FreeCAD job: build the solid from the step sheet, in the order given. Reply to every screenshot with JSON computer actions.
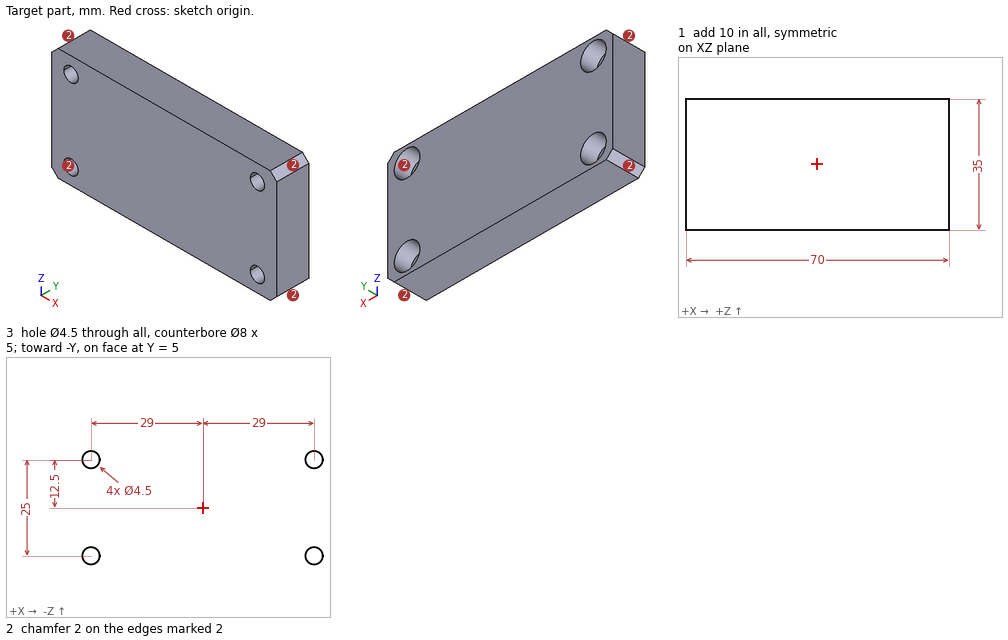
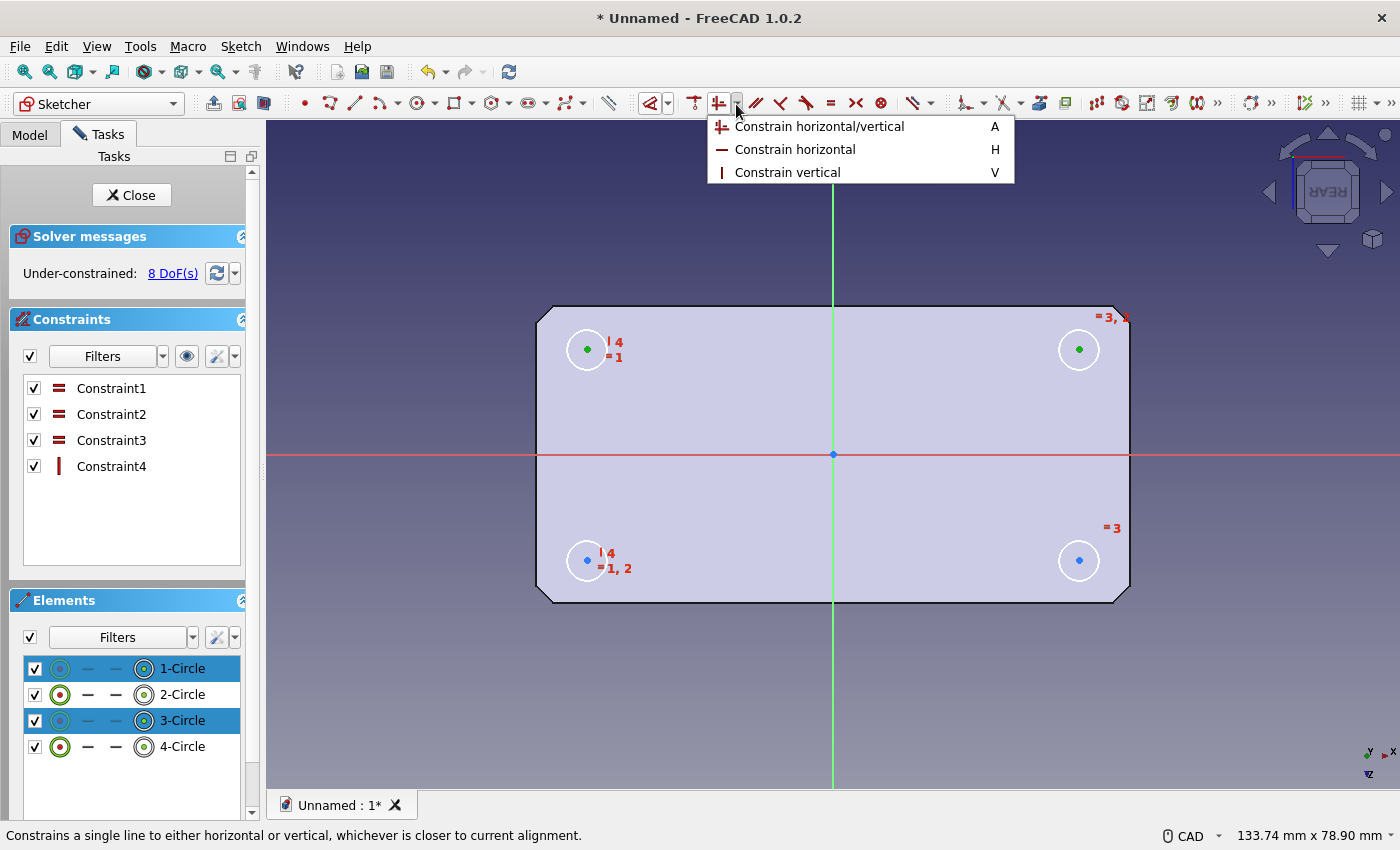
{"action": "left_click", "coordinate": [861, 150]}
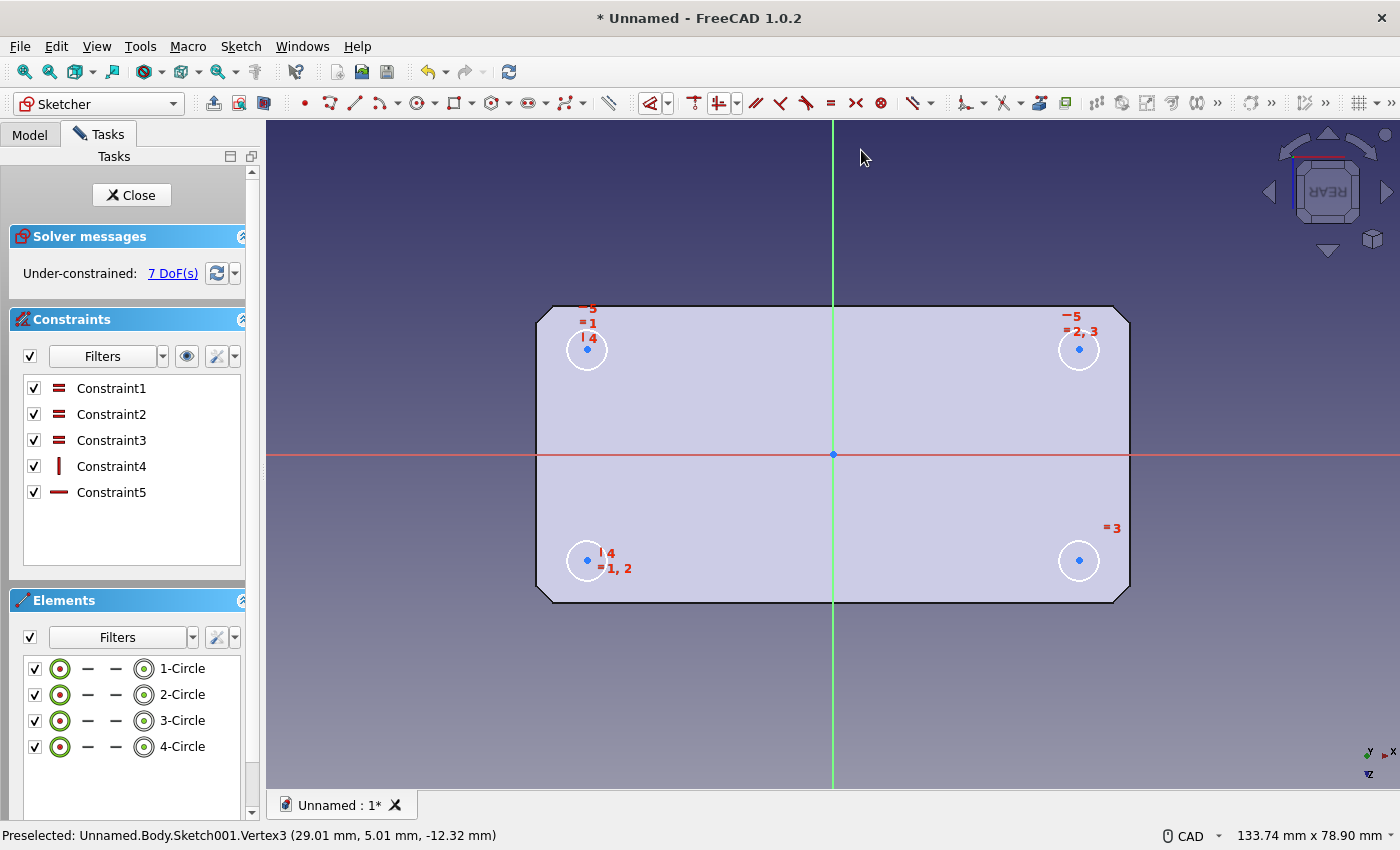
{"action": "left_click", "coordinate": [1079, 350]}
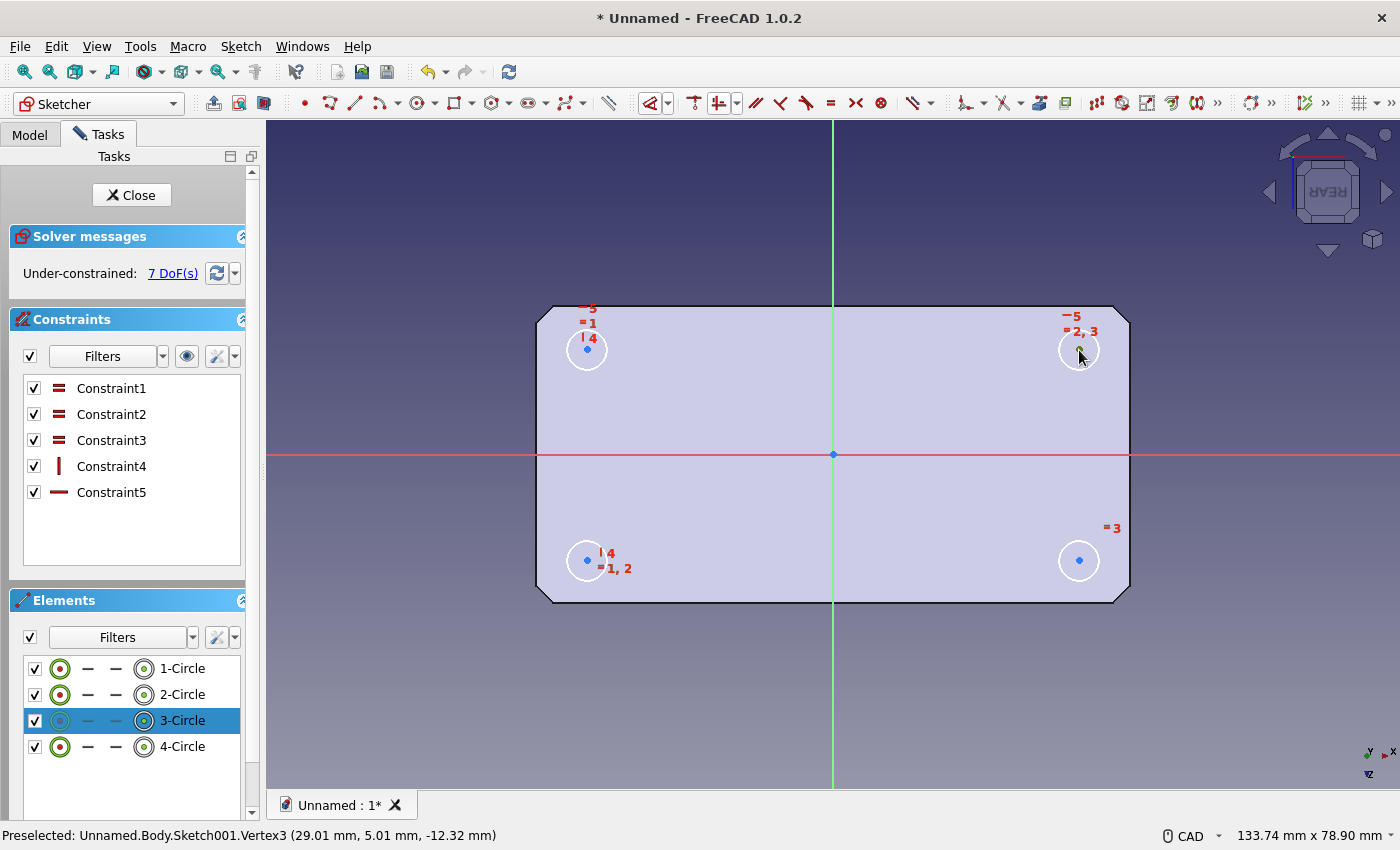
{"action": "left_click", "coordinate": [1079, 561]}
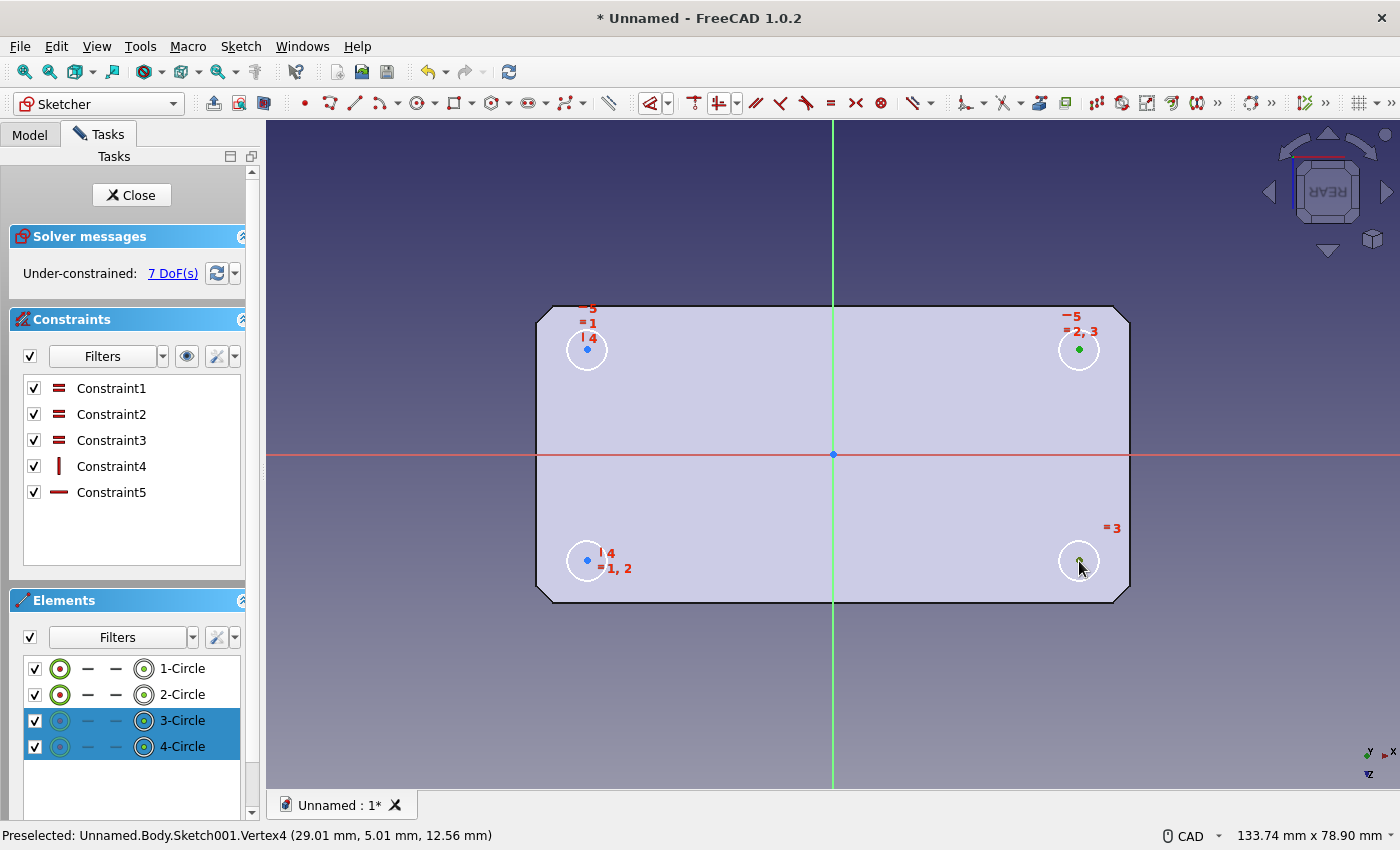
{"action": "left_click", "coordinate": [736, 104]}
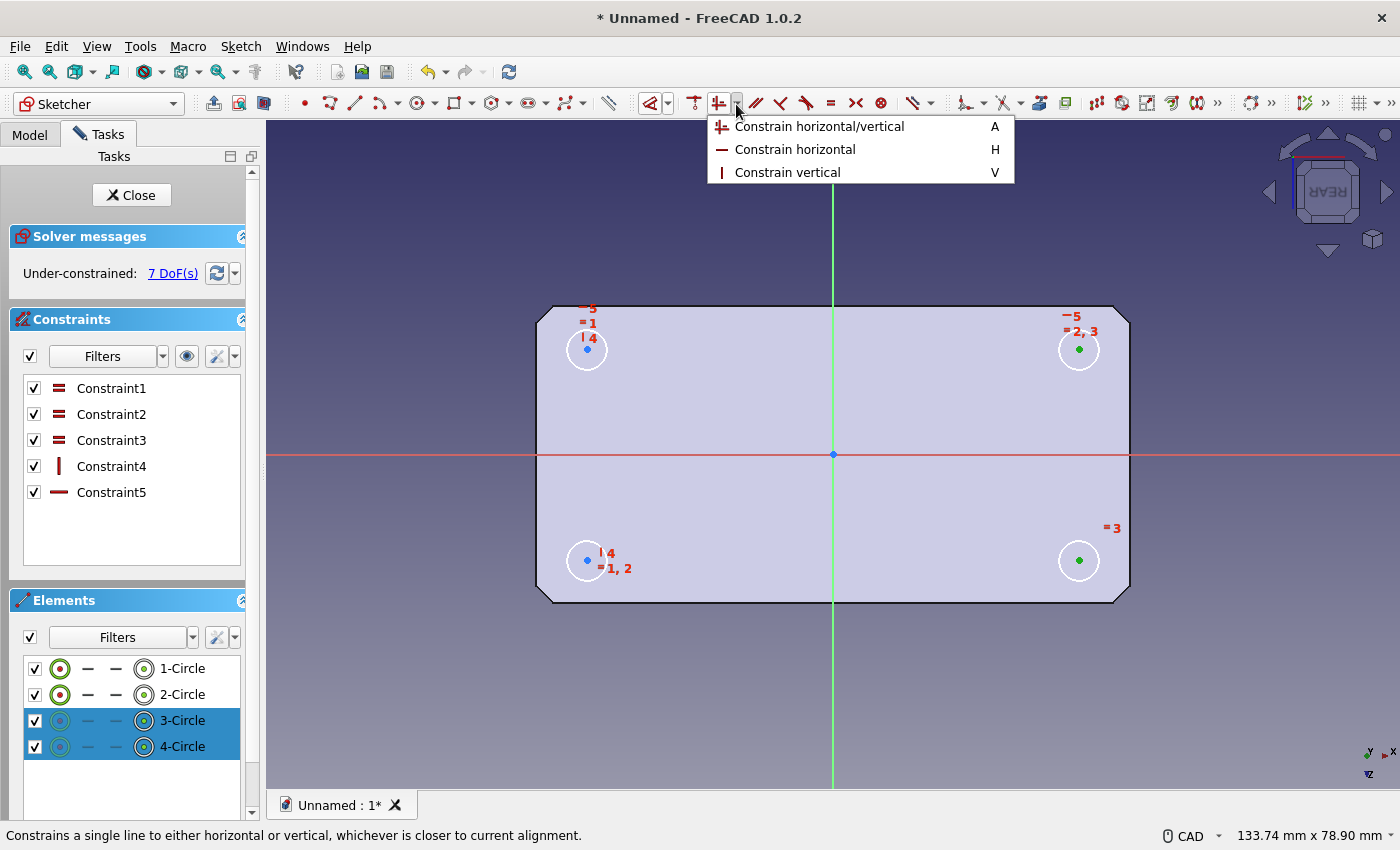
{"action": "left_click", "coordinate": [861, 172]}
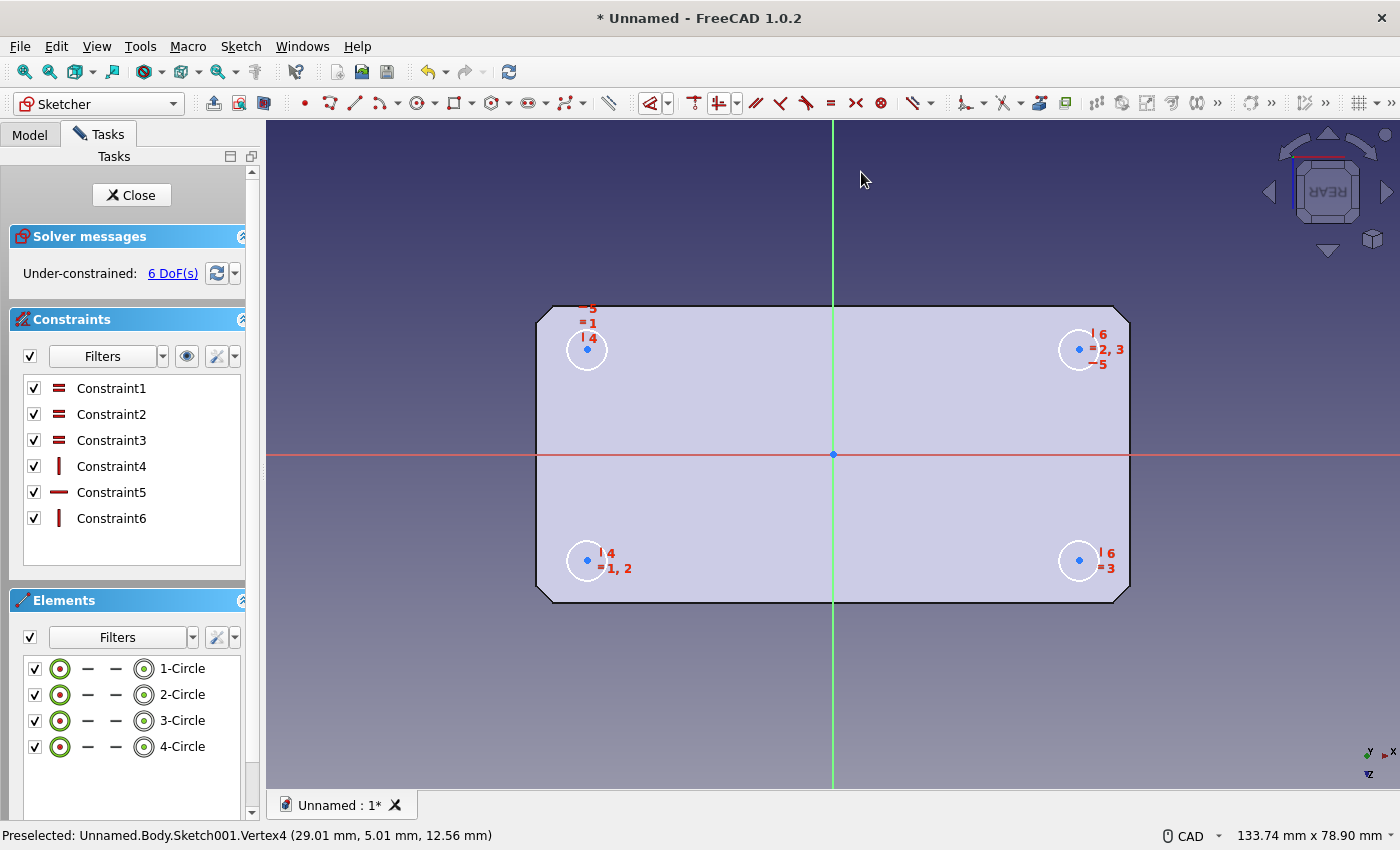
{"action": "left_click", "coordinate": [587, 561]}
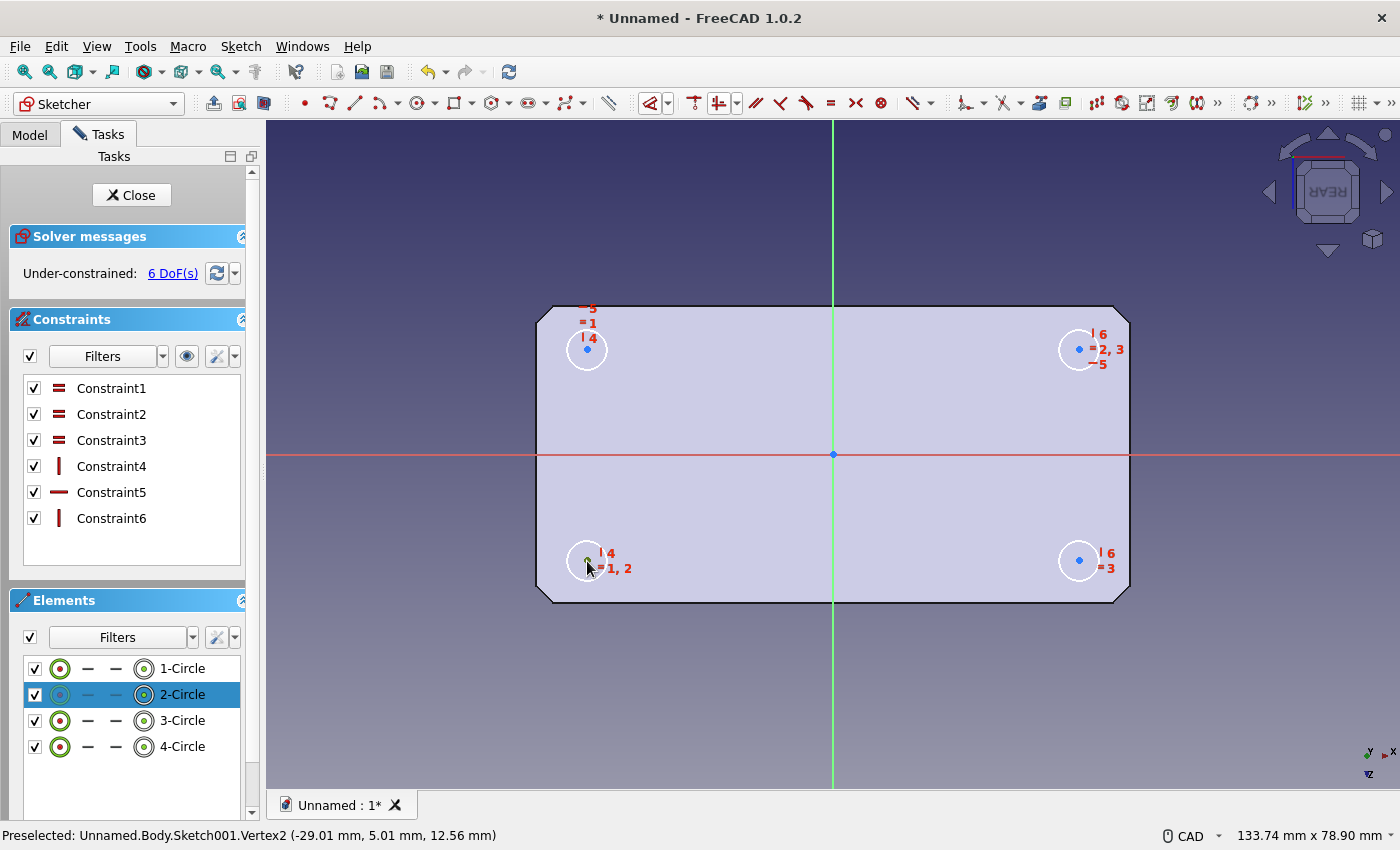
{"action": "left_click", "coordinate": [1079, 561]}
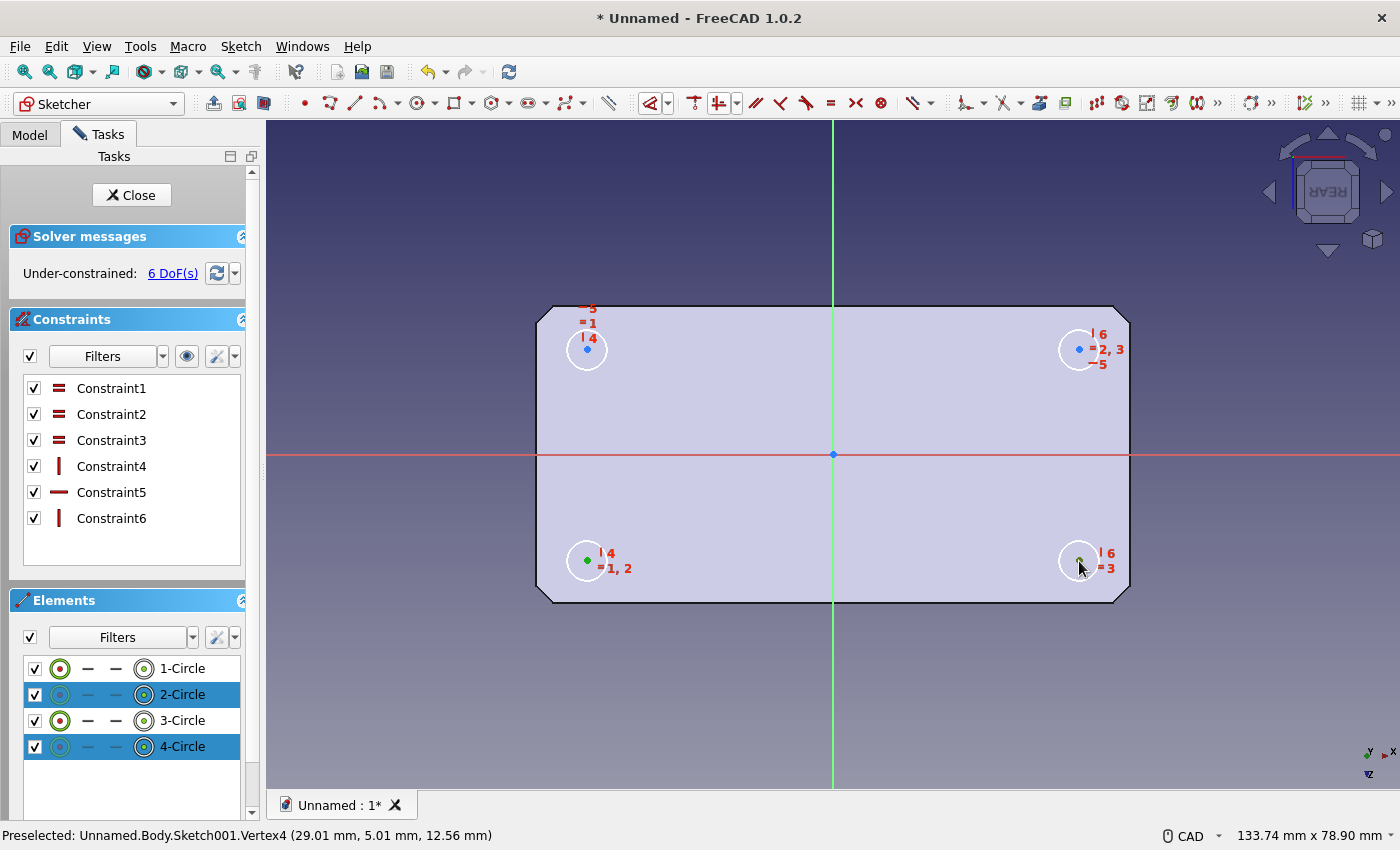
{"action": "left_click", "coordinate": [736, 104]}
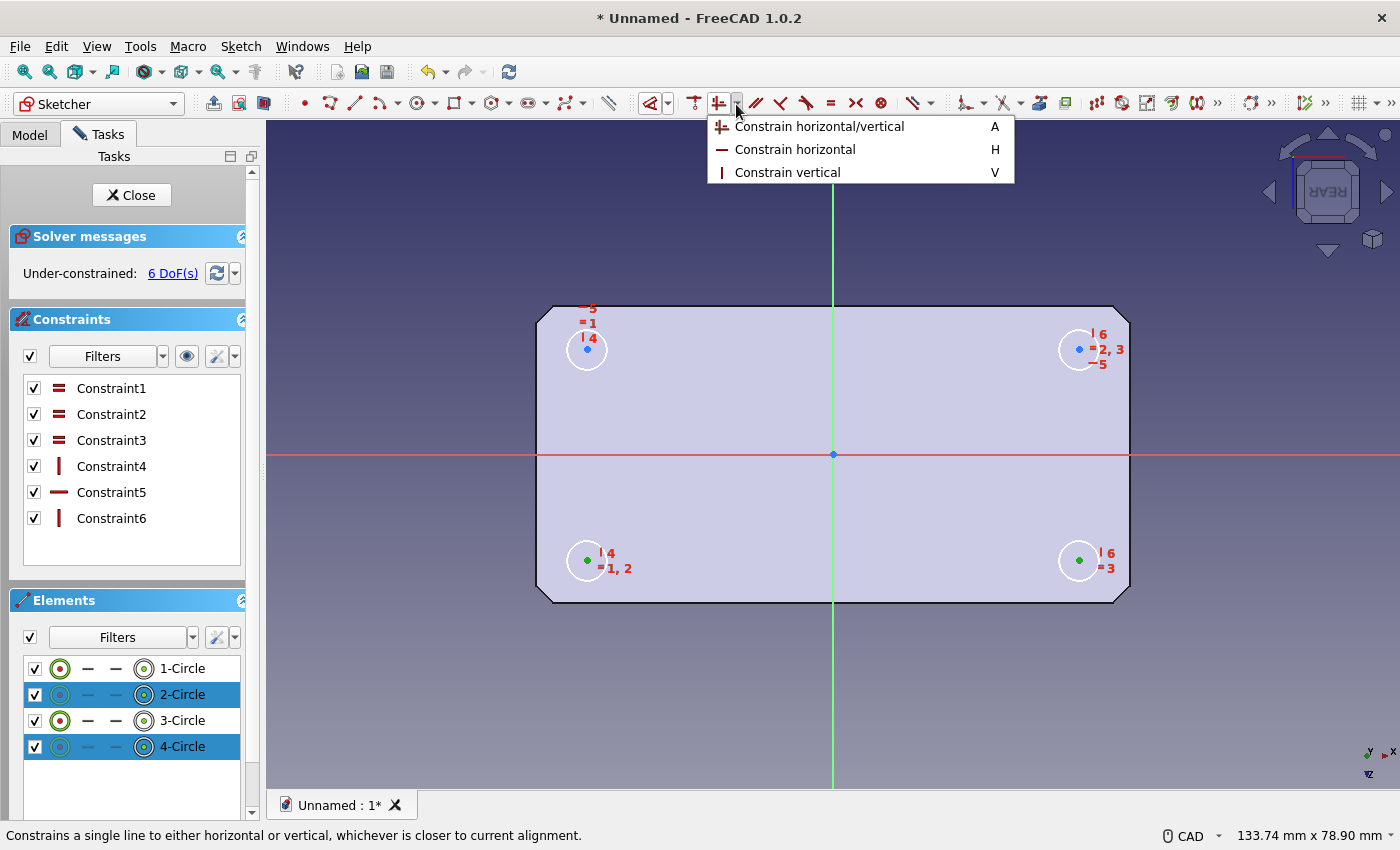
{"action": "left_click", "coordinate": [861, 150]}